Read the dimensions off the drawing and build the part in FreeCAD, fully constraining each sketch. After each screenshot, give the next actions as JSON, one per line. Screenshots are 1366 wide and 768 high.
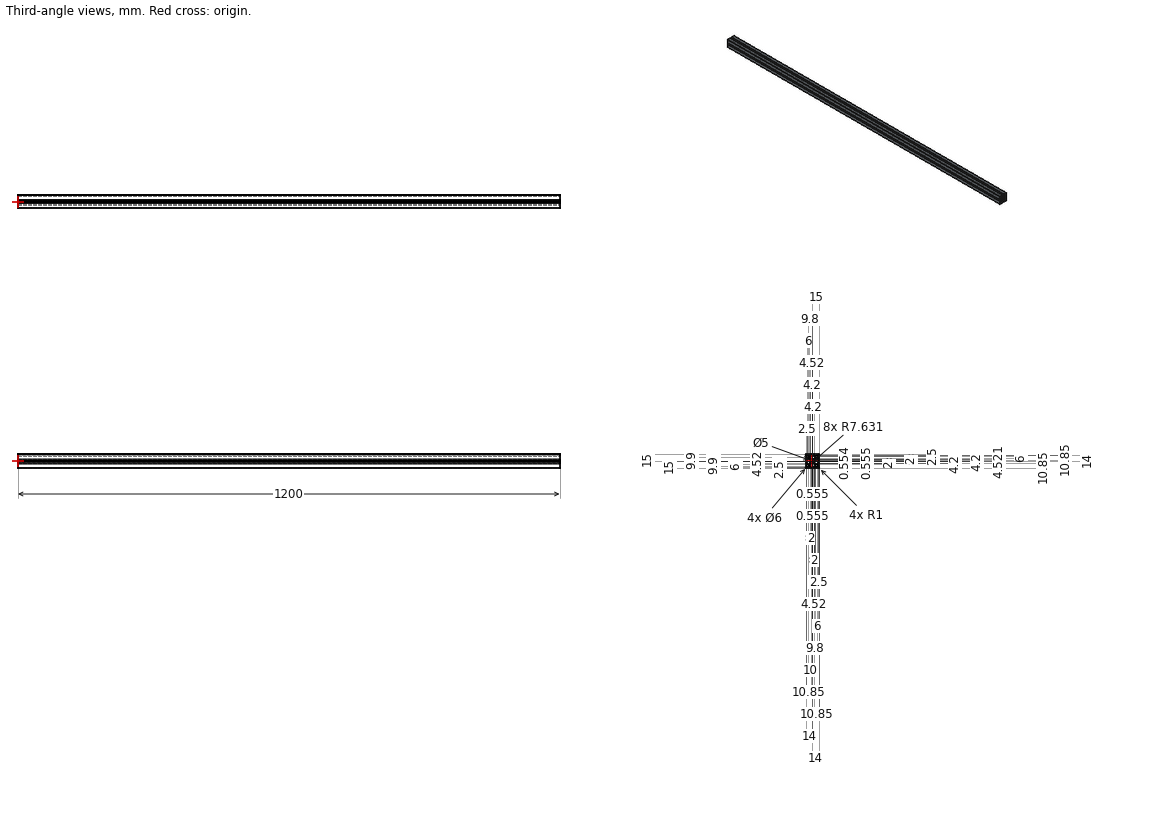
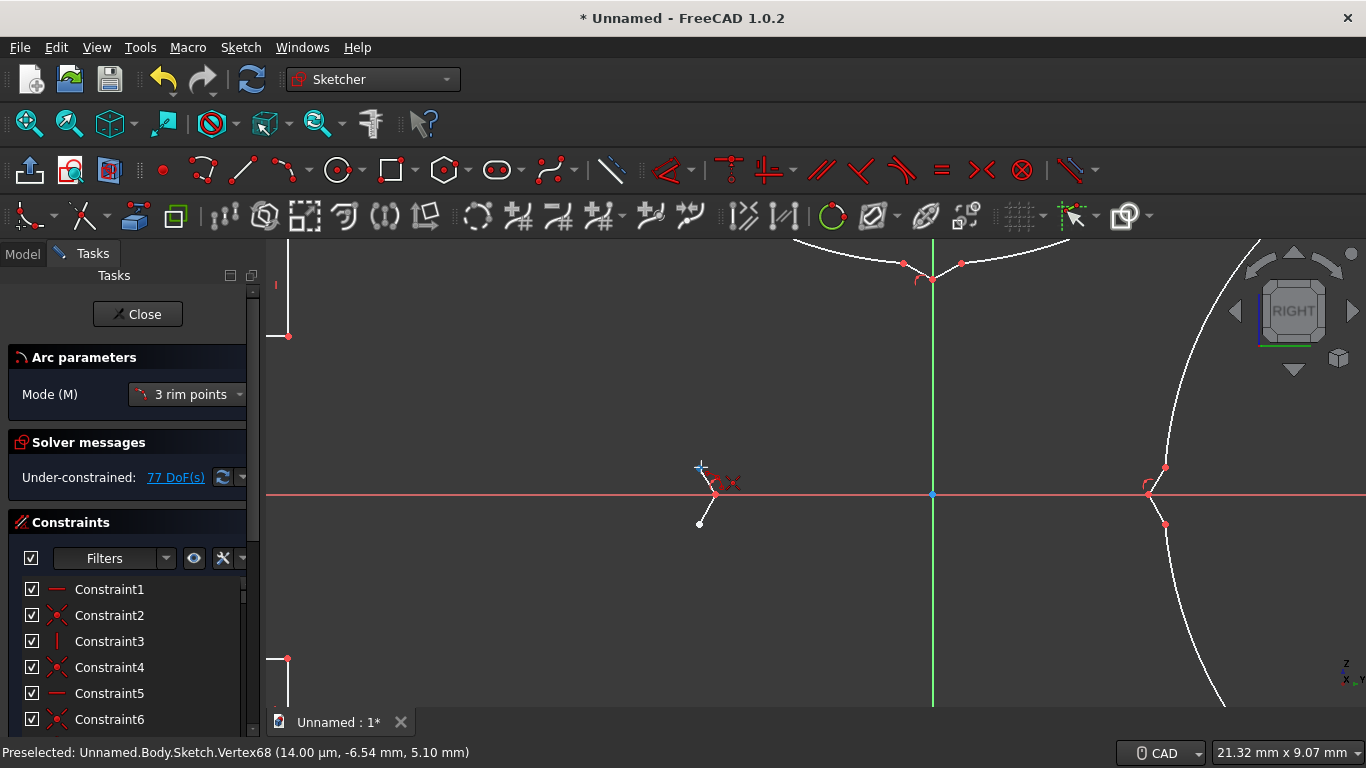
{"action": "left_click", "coordinate": [699, 468]}
{"action": "left_click", "coordinate": [668, 339]}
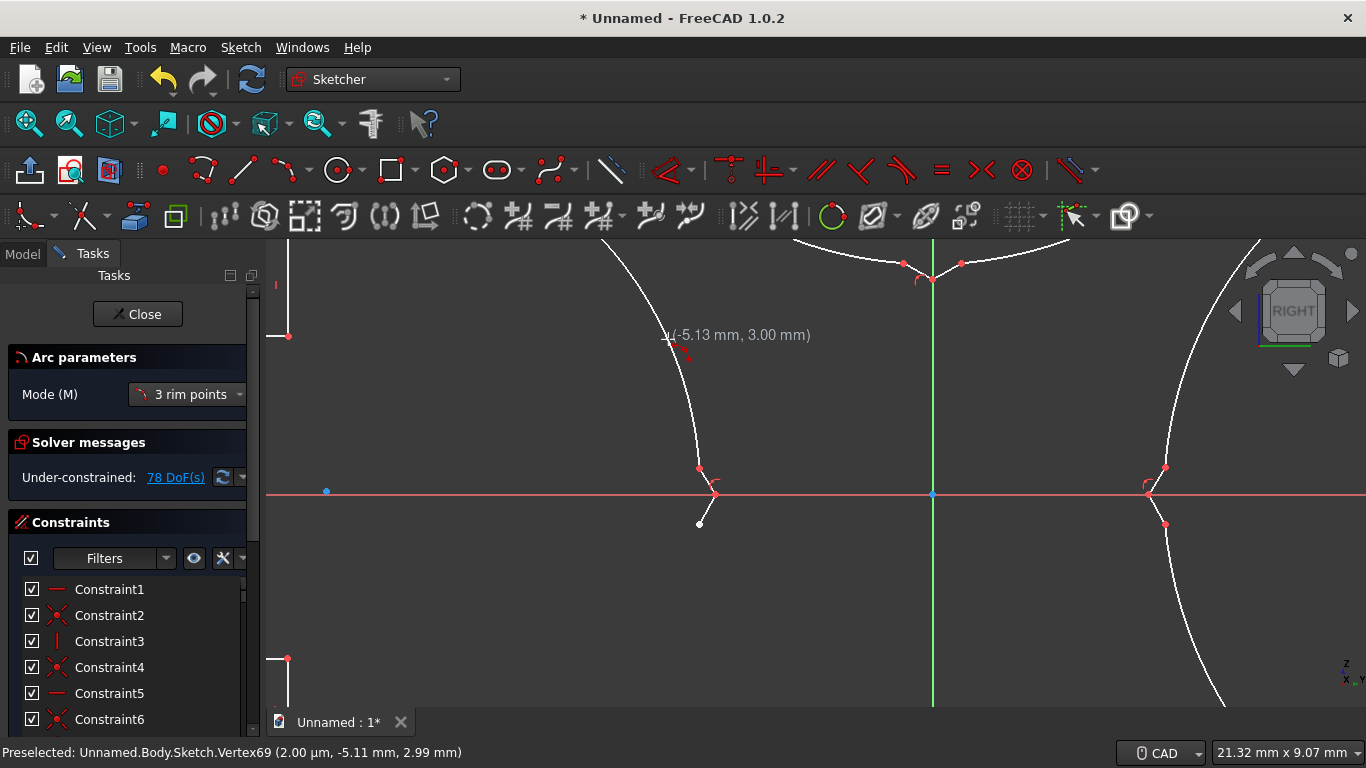
{"action": "left_click", "coordinate": [699, 525]}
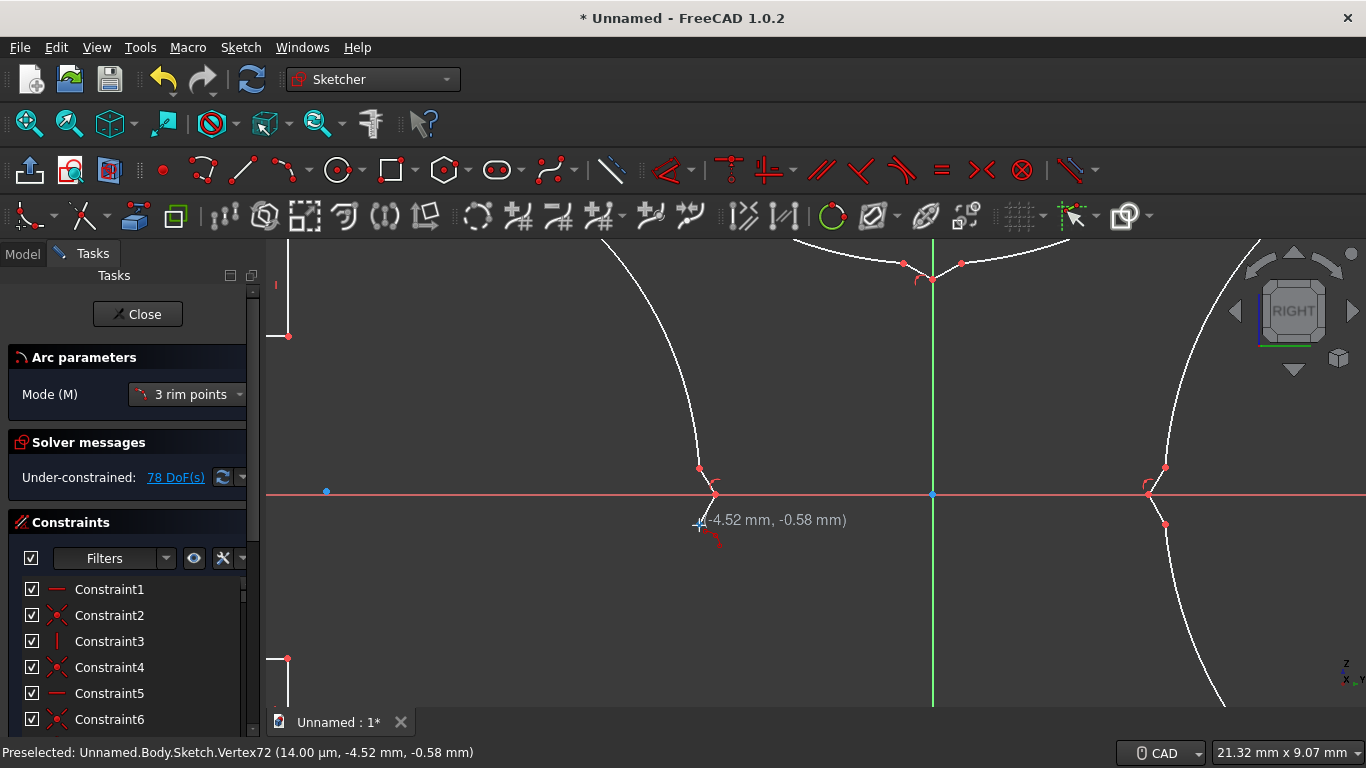
{"action": "scroll", "coordinate": [701, 467], "scroll_direction": "down", "scroll_amount": 8}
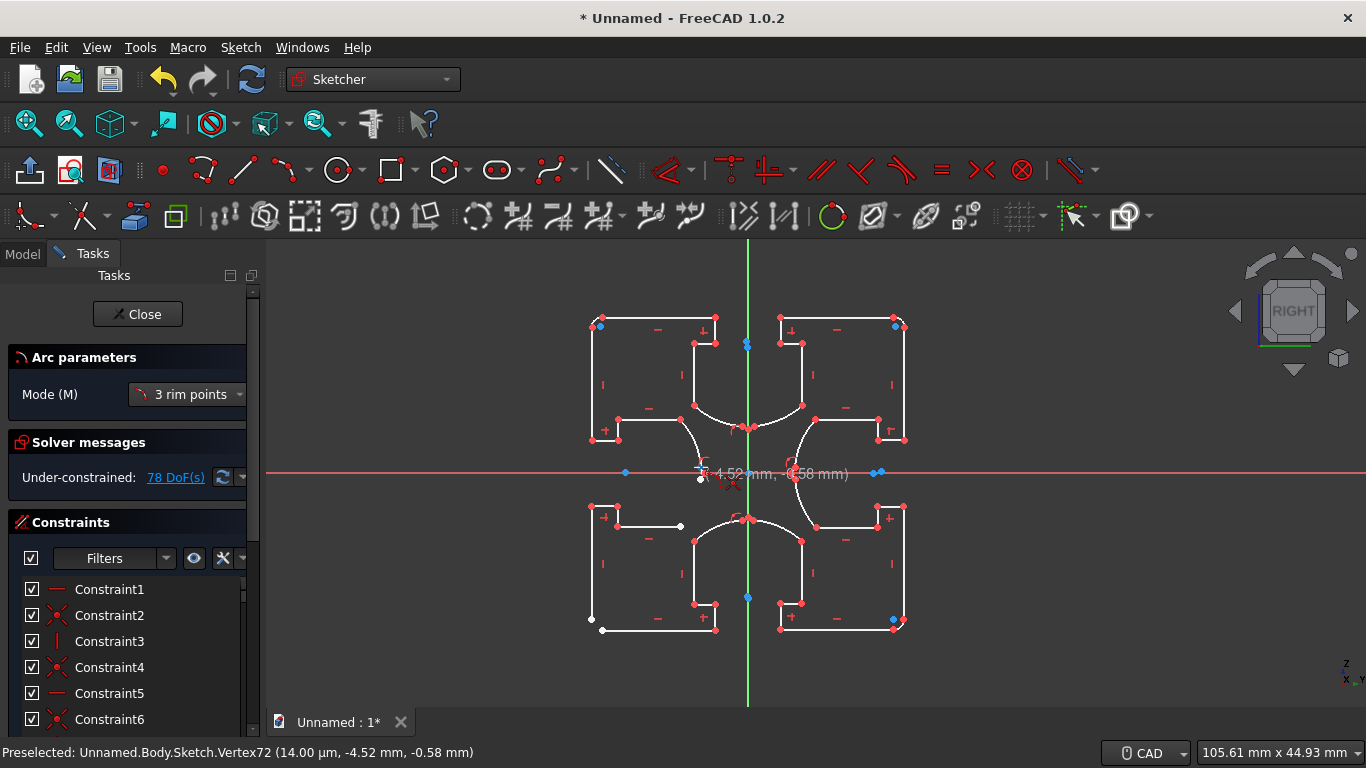
{"action": "left_click", "coordinate": [680, 527]}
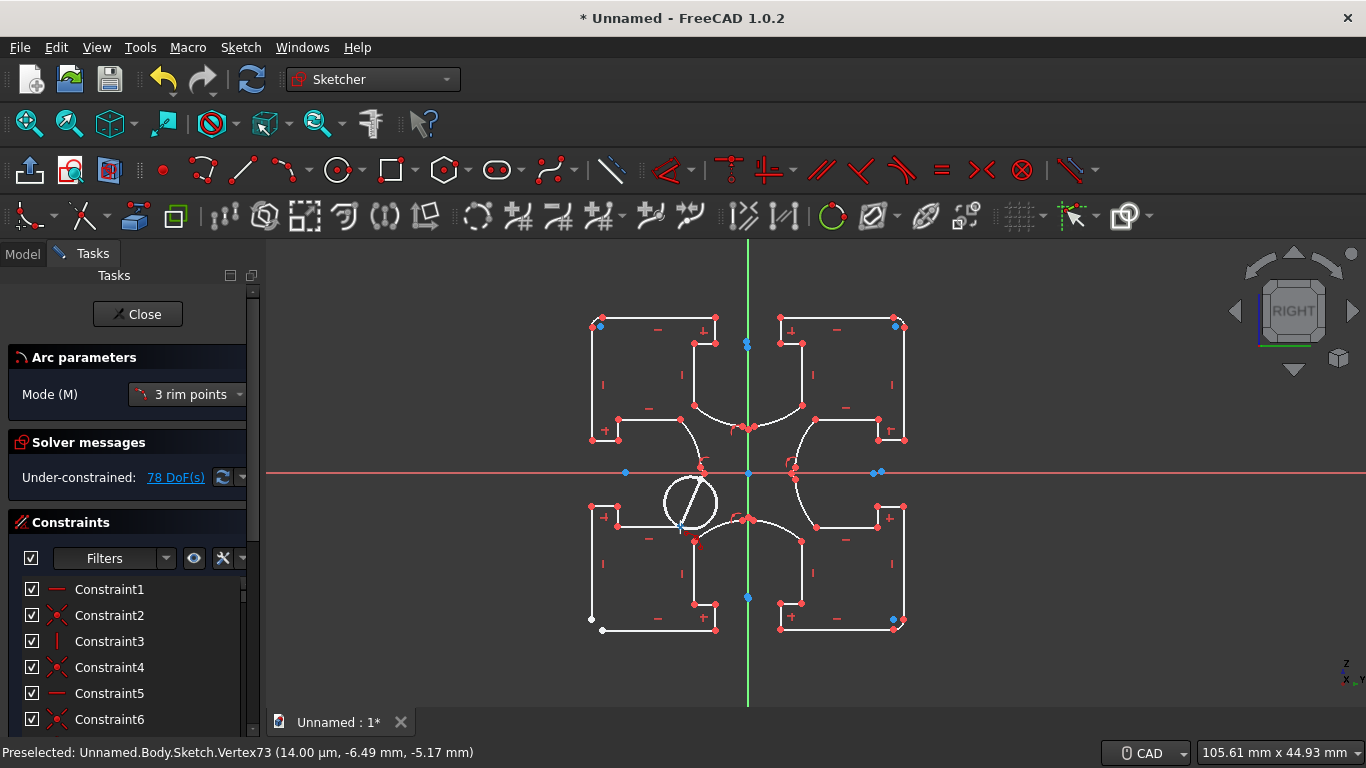
{"action": "scroll", "coordinate": [695, 504], "scroll_direction": "up", "scroll_amount": 7}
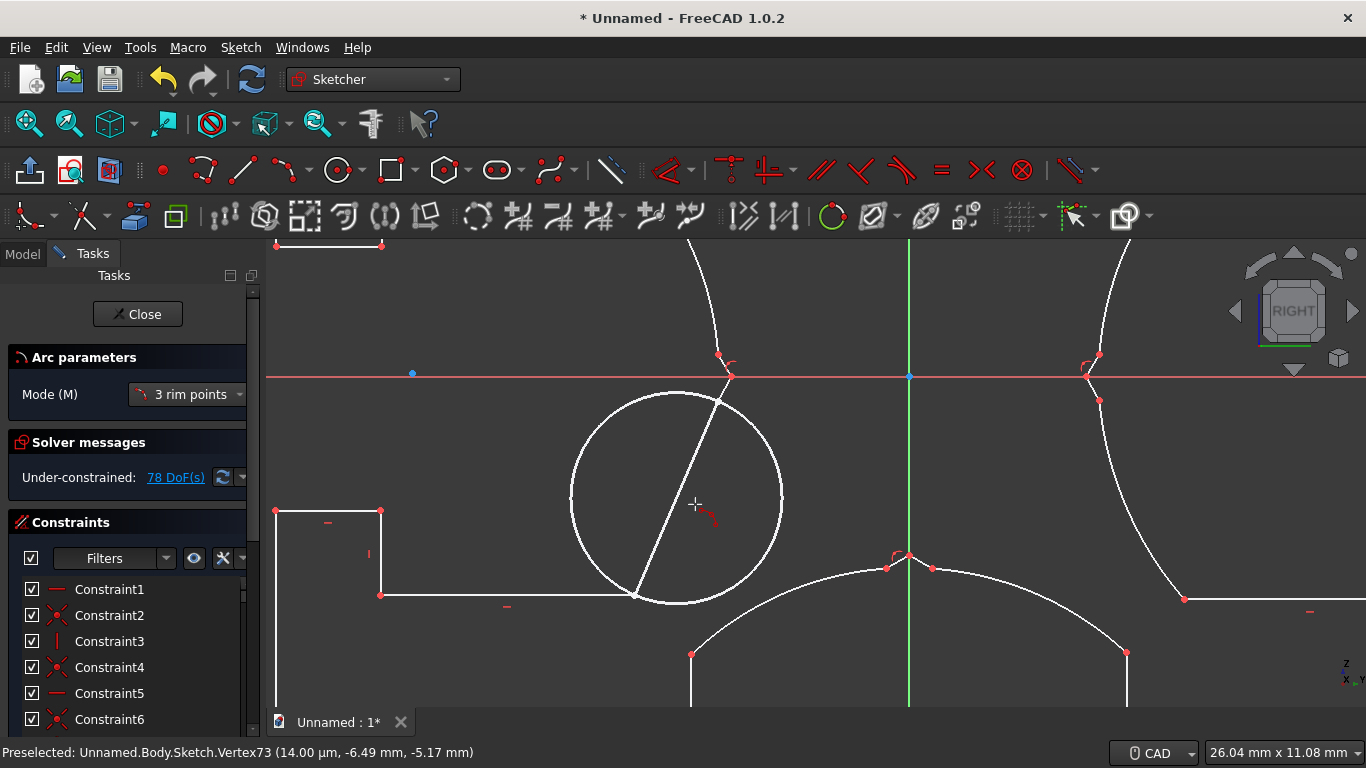
{"action": "left_click", "coordinate": [693, 504]}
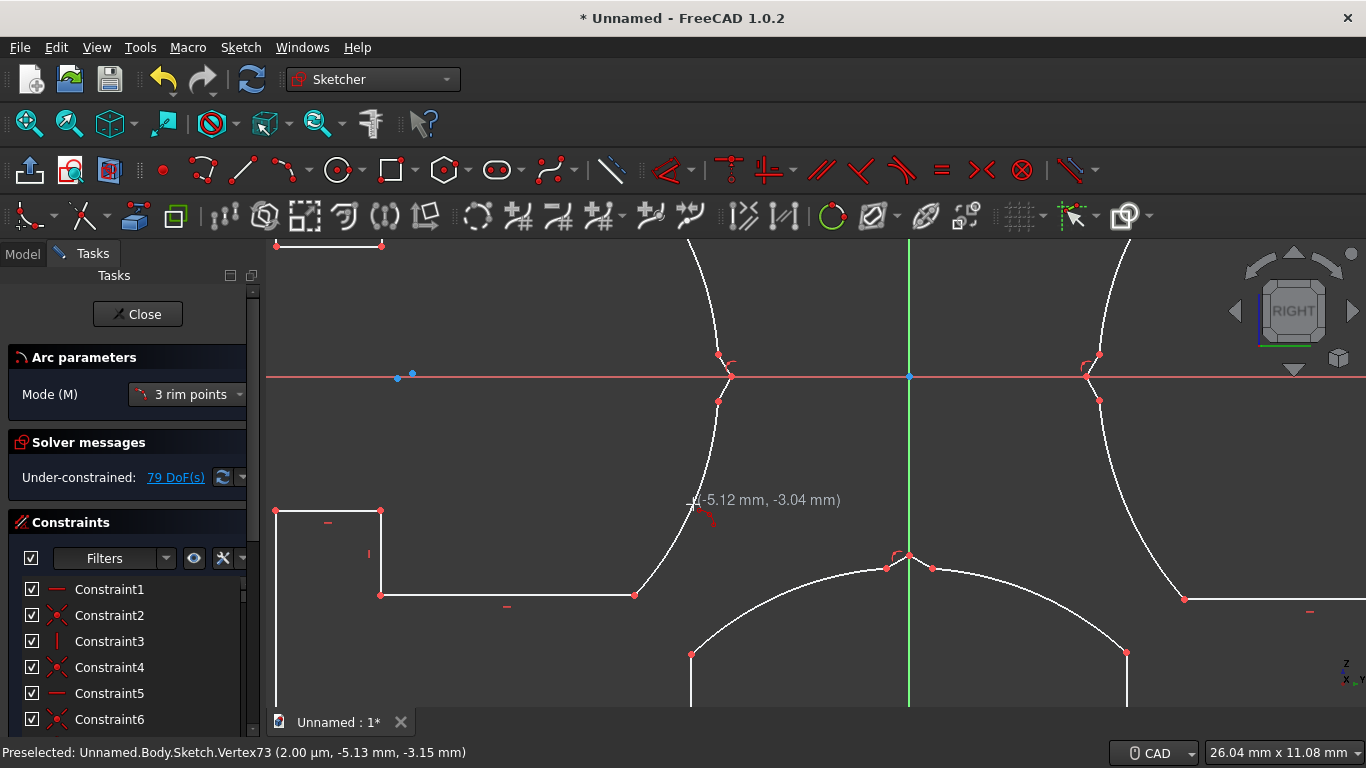
{"action": "scroll", "coordinate": [695, 505], "scroll_direction": "down", "scroll_amount": 7}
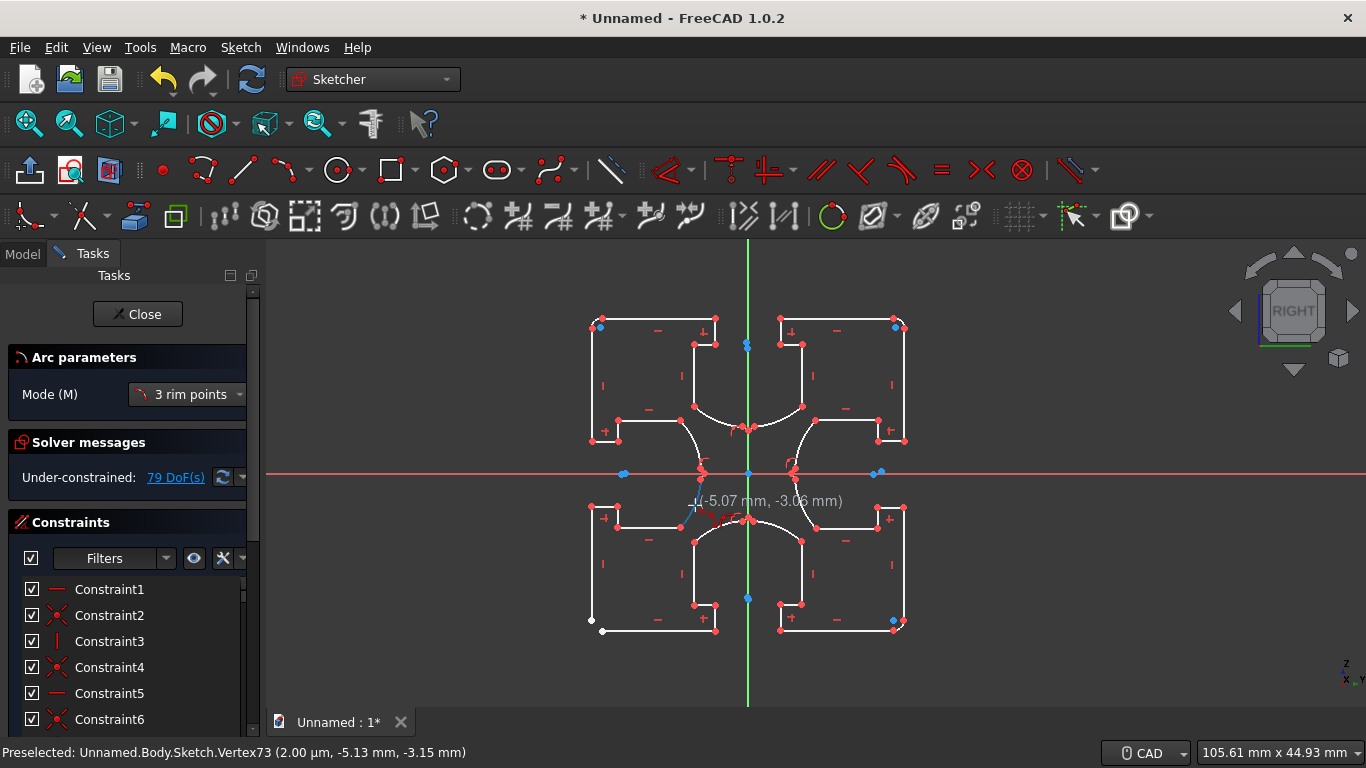
{"action": "left_click", "coordinate": [592, 621]}
{"action": "left_click", "coordinate": [602, 631]}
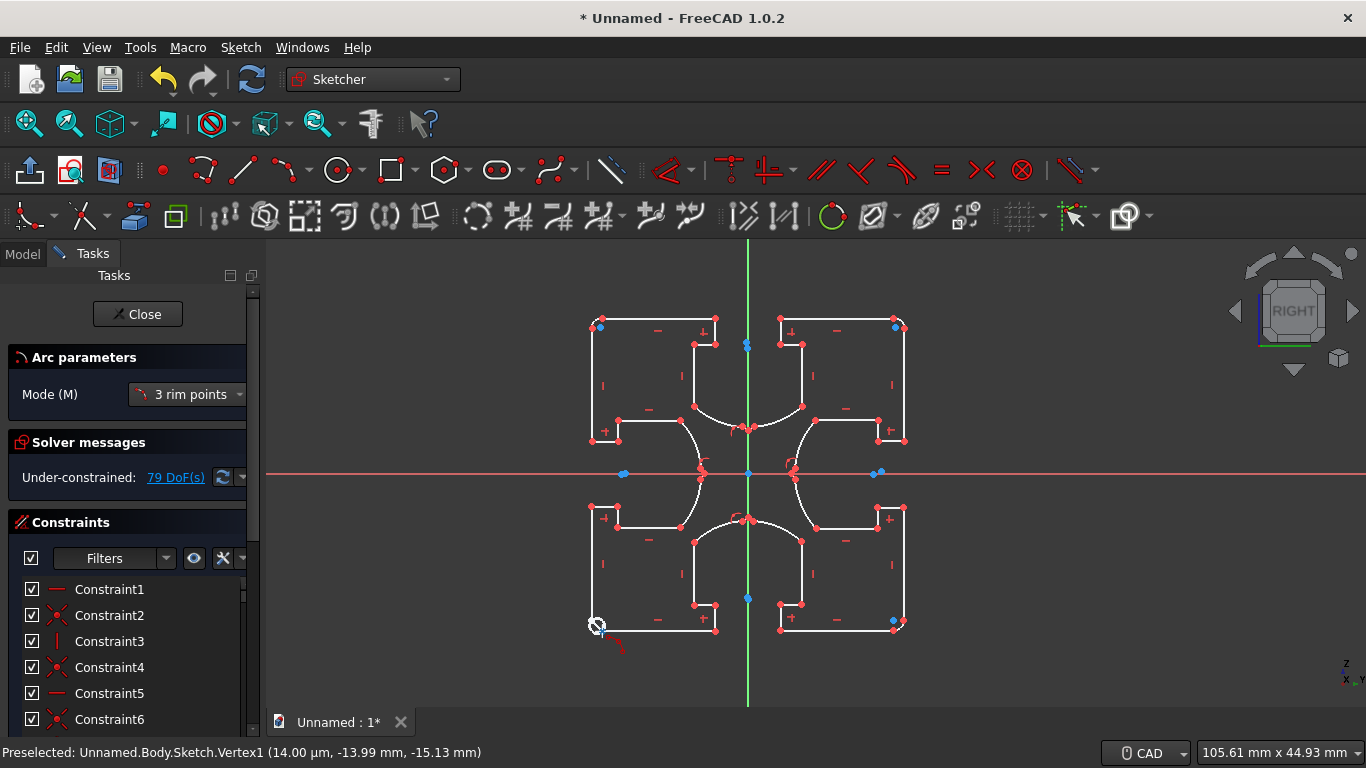
{"action": "scroll", "coordinate": [595, 627], "scroll_direction": "up", "scroll_amount": 9}